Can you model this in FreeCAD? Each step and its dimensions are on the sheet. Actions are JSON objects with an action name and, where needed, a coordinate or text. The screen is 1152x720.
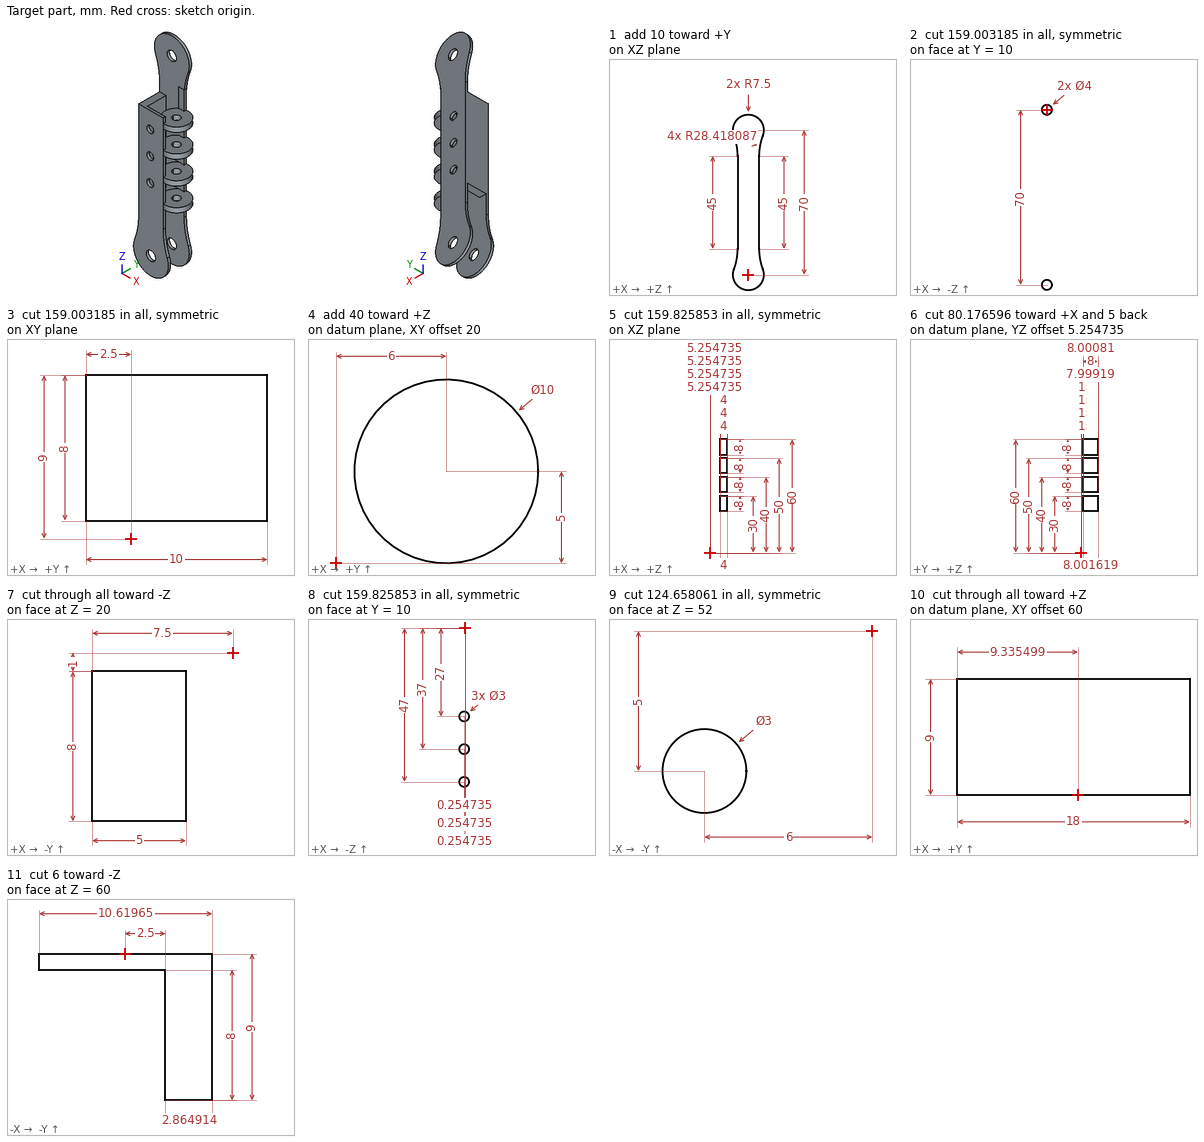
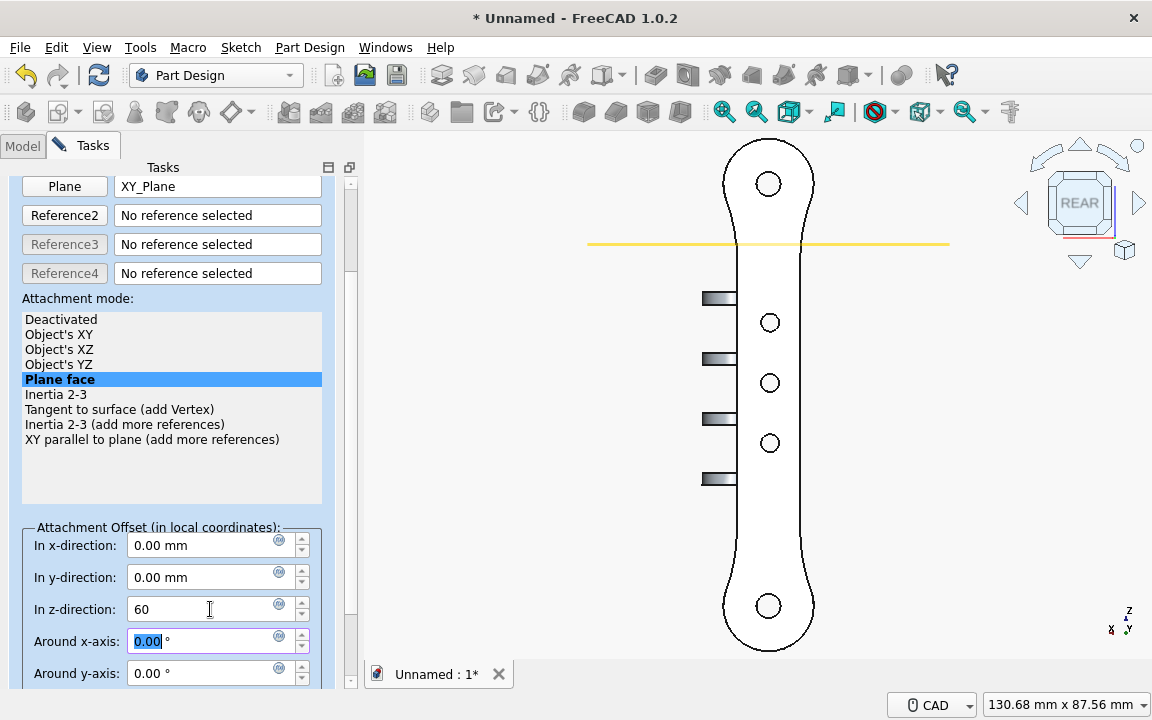
{"action": "scroll", "coordinate": [351, 432], "scroll_direction": "up", "scroll_amount": 3}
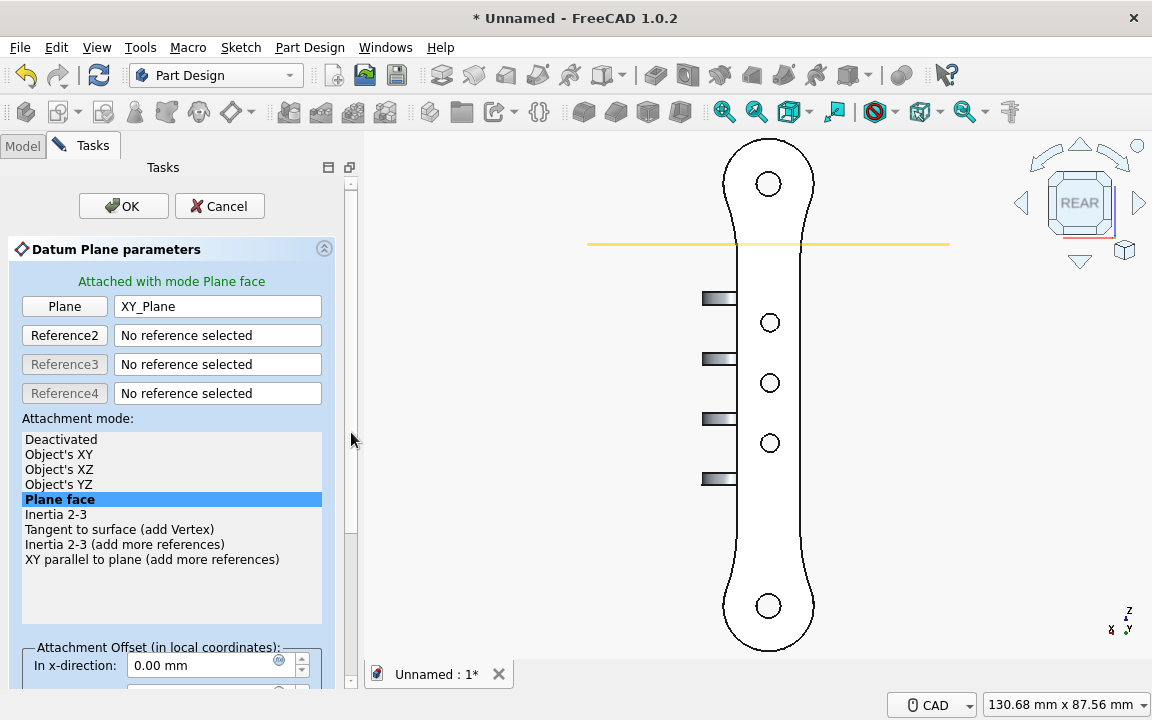
{"action": "left_click", "coordinate": [124, 206]}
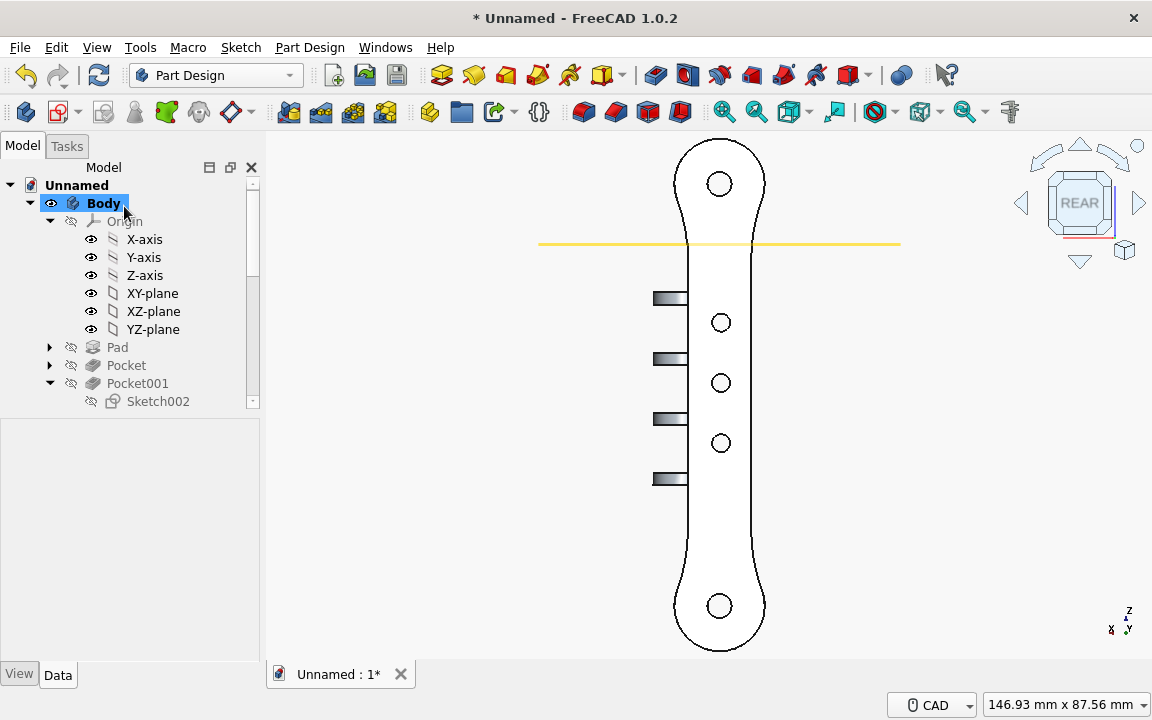
{"action": "scroll", "coordinate": [100, 289], "scroll_direction": "down", "scroll_amount": 3}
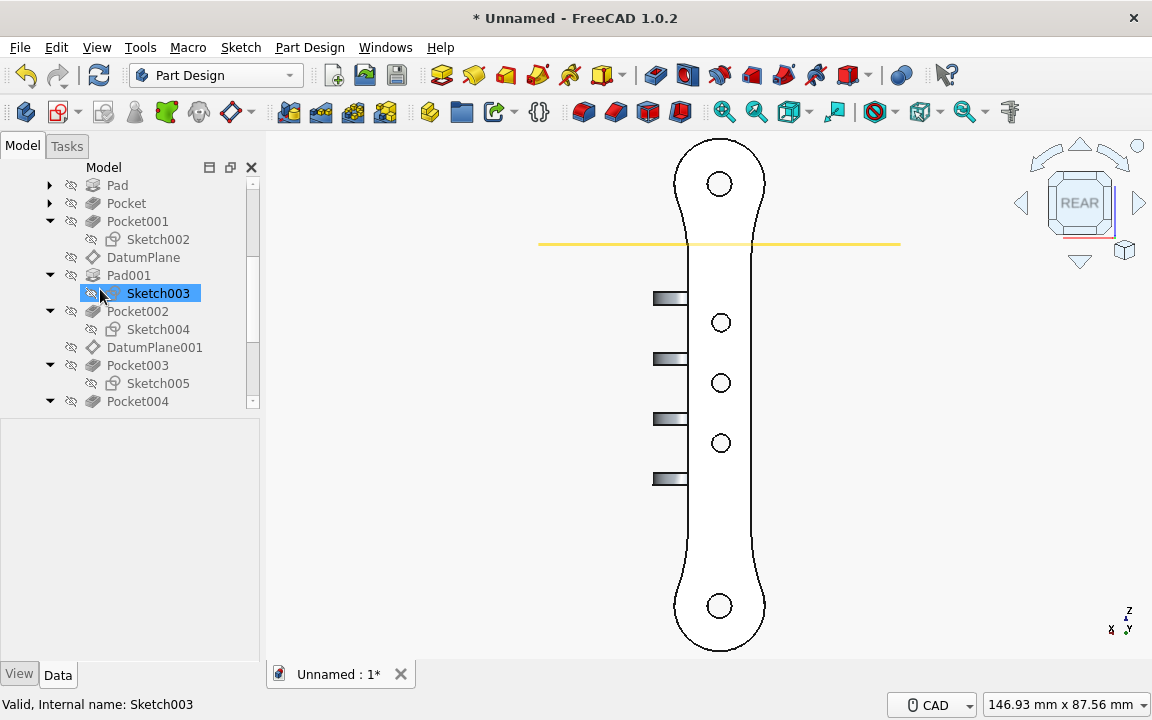
{"action": "scroll", "coordinate": [140, 289], "scroll_direction": "up", "scroll_amount": 15}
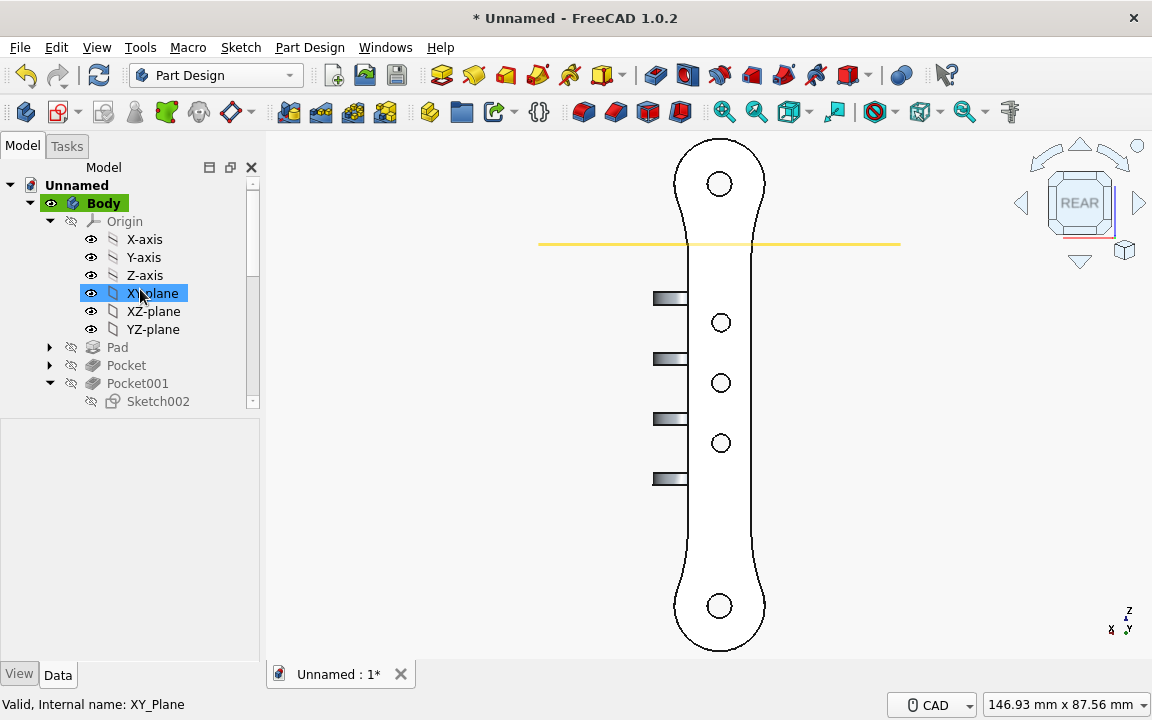
{"action": "scroll", "coordinate": [100, 289], "scroll_direction": "down", "scroll_amount": 6}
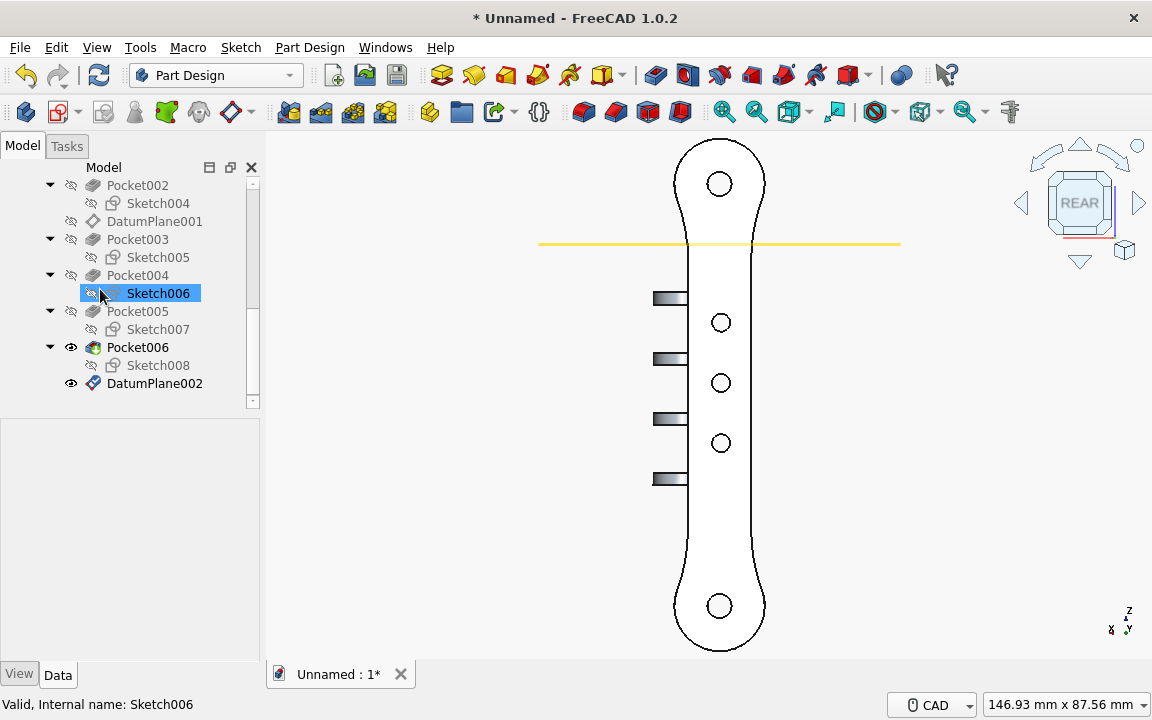
{"action": "left_click", "coordinate": [116, 383]}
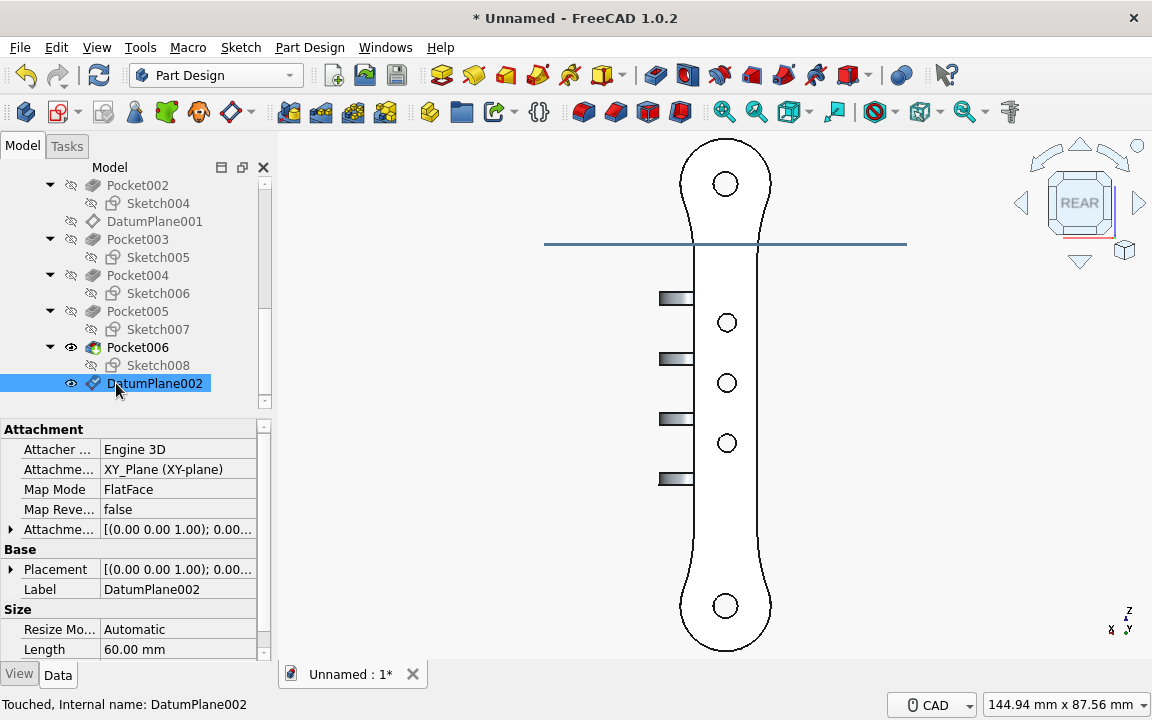
{"action": "left_click", "coordinate": [58, 112]}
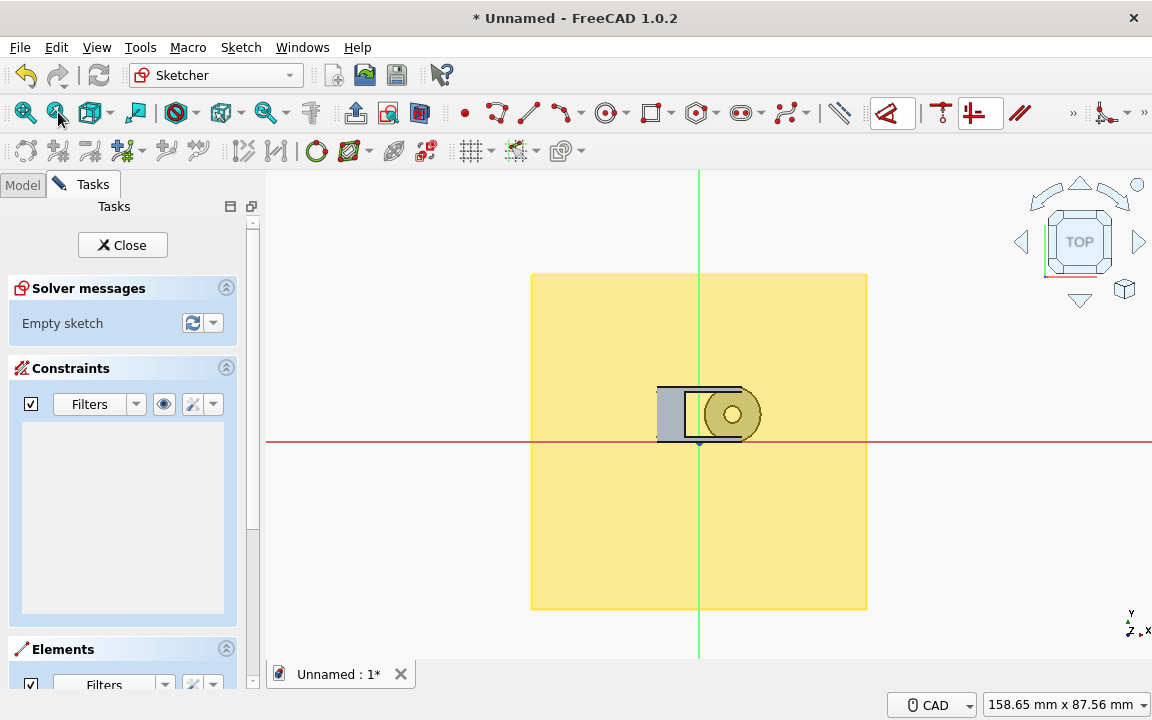
{"action": "left_click", "coordinate": [420, 114]}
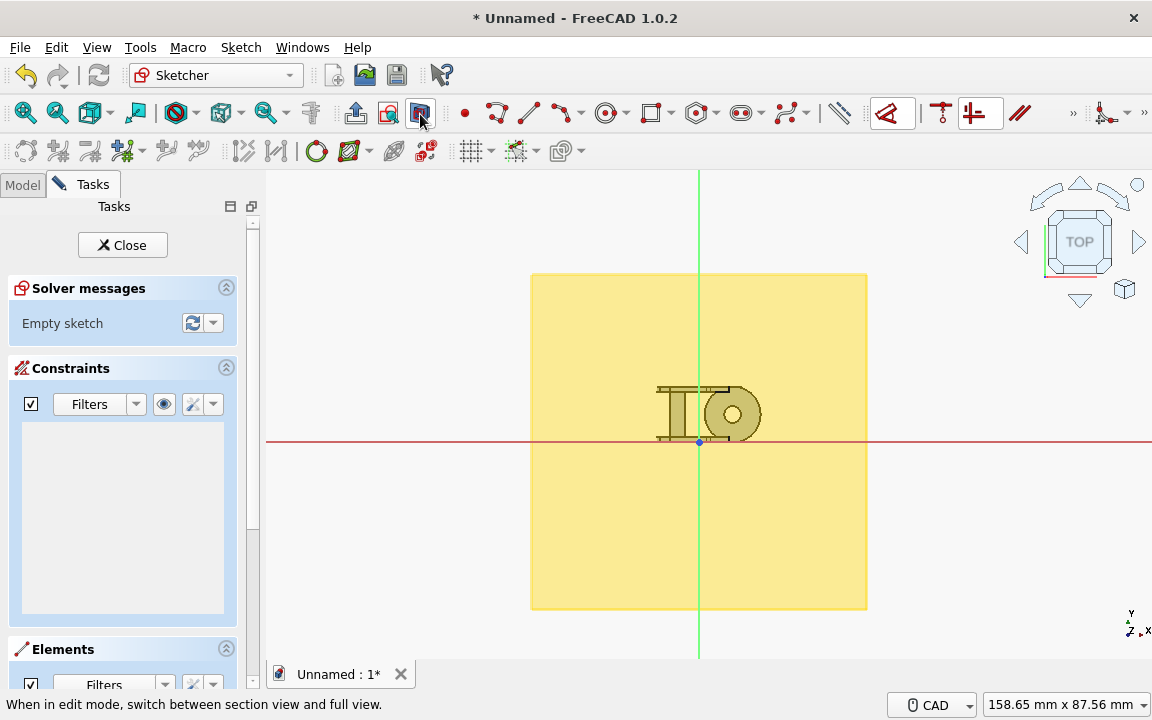
{"action": "scroll", "coordinate": [712, 418], "scroll_direction": "up", "scroll_amount": 8}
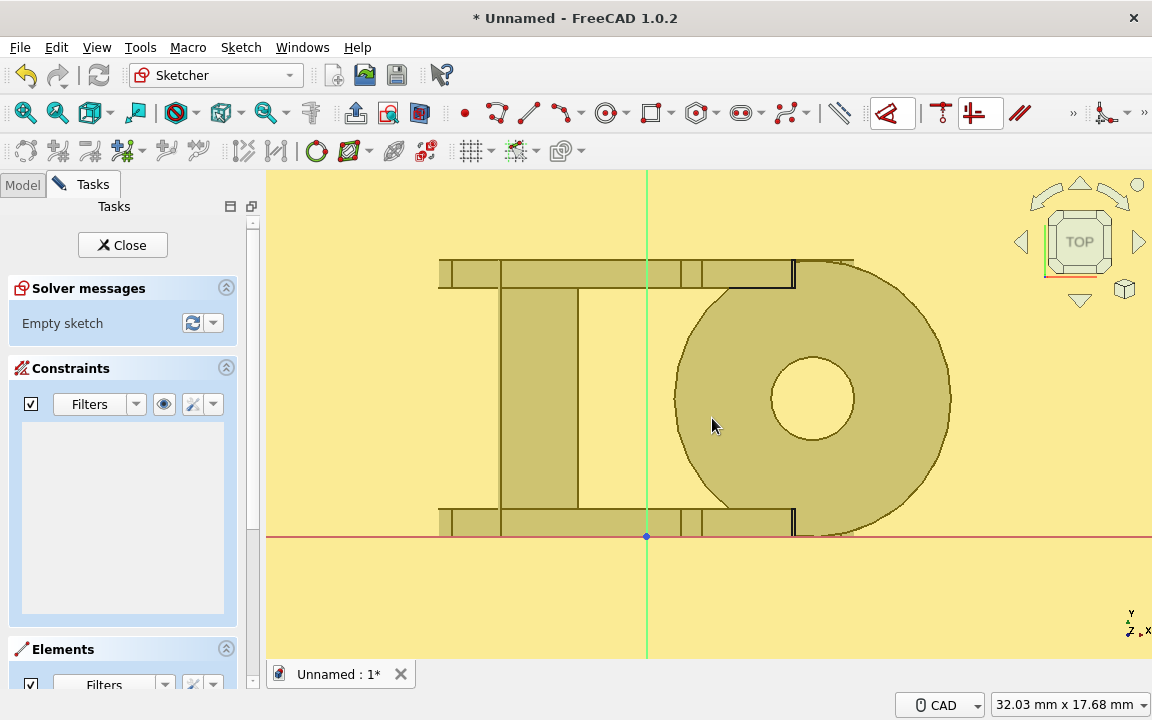
{"action": "left_click", "coordinate": [652, 114]}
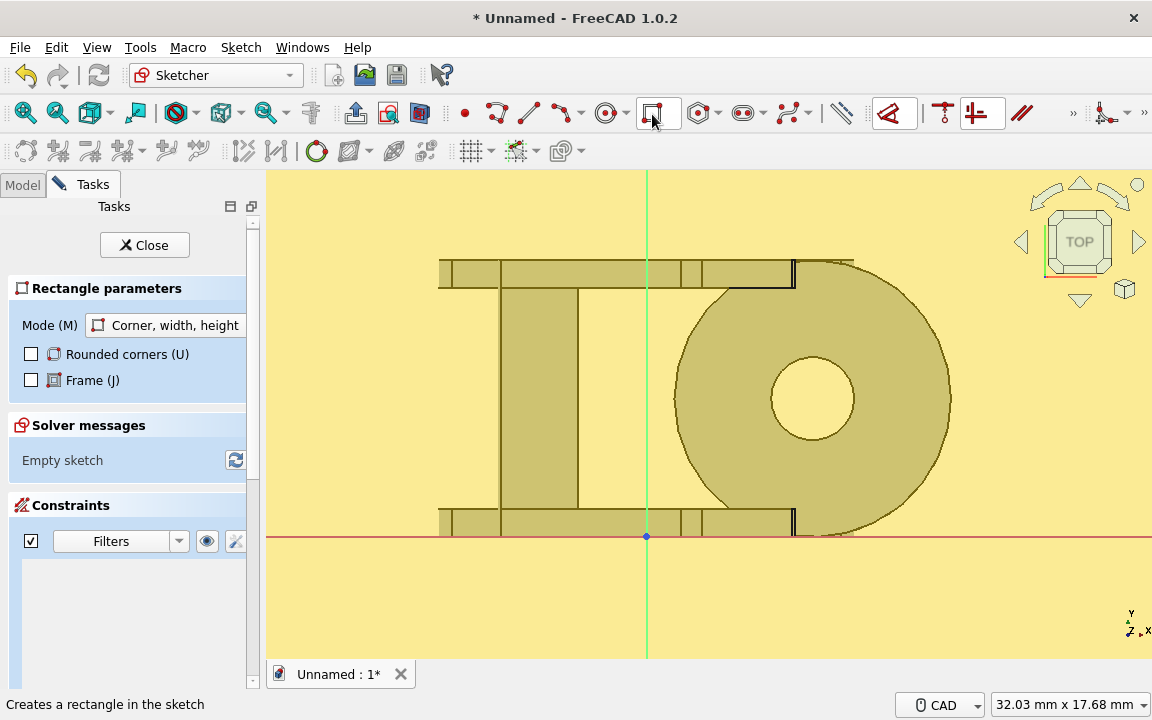
{"action": "left_click", "coordinate": [389, 288]}
{"action": "left_click", "coordinate": [886, 537]}
{"action": "key", "text": "Escape"}